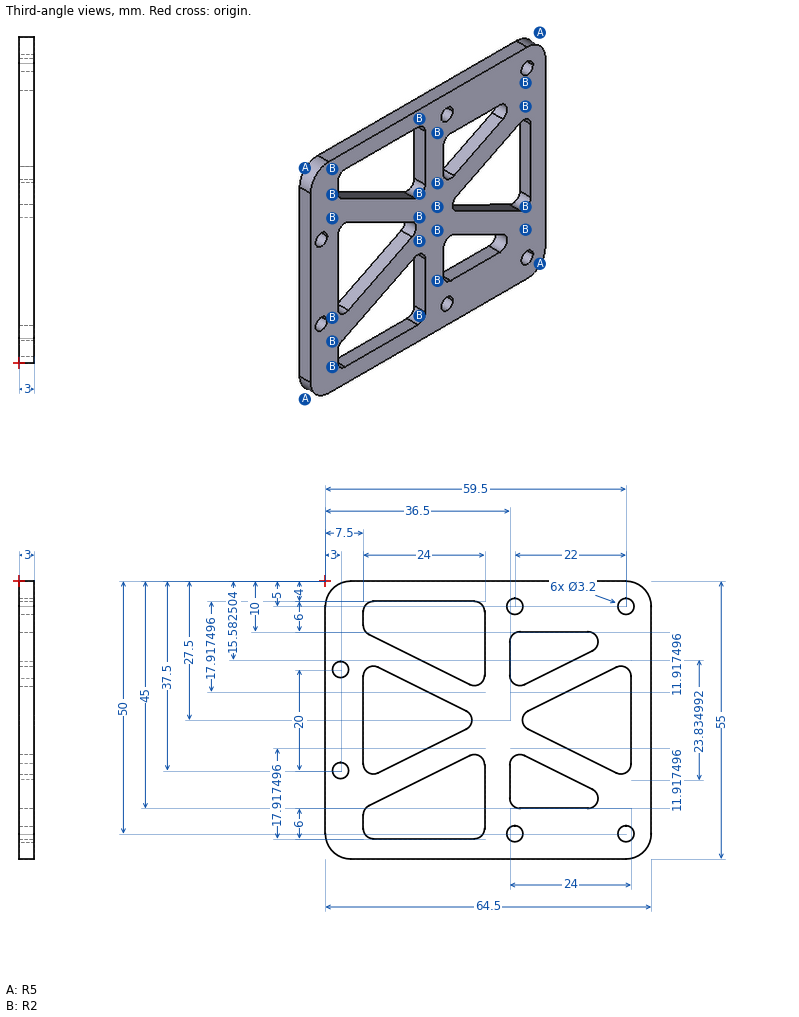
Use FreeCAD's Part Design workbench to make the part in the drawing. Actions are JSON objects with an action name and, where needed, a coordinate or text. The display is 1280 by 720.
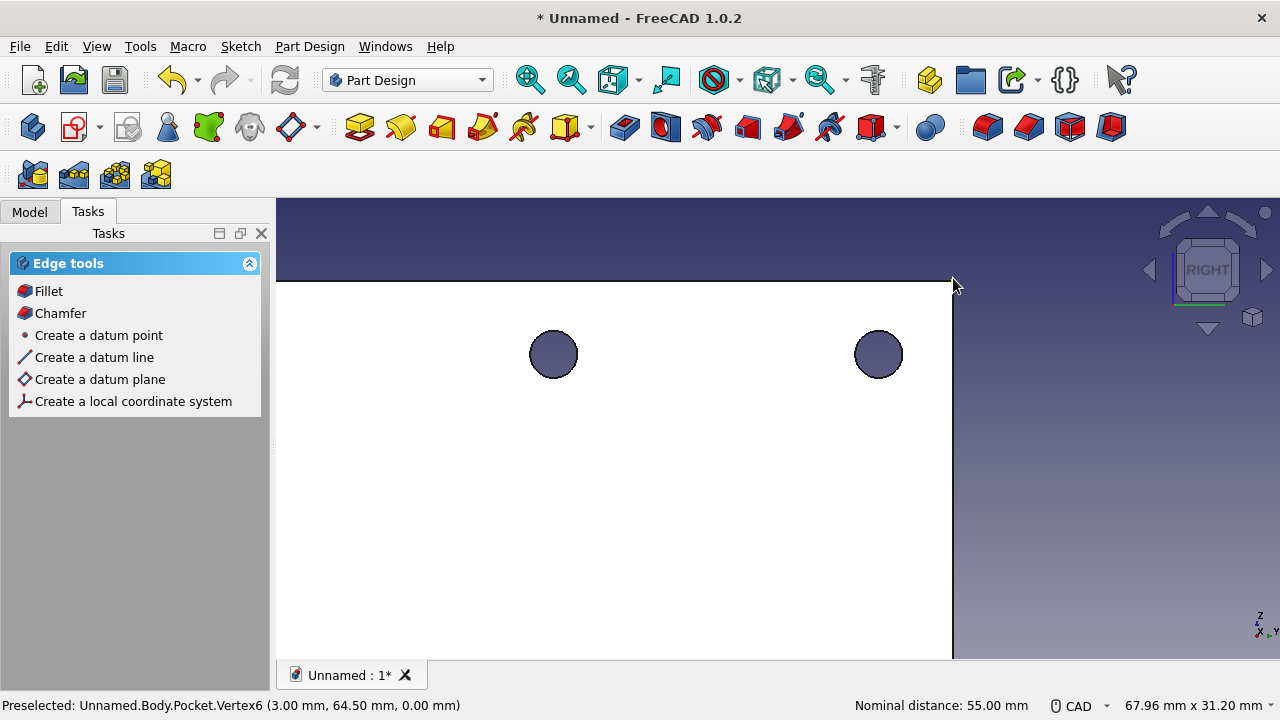
{"action": "left_click", "coordinate": [531, 80]}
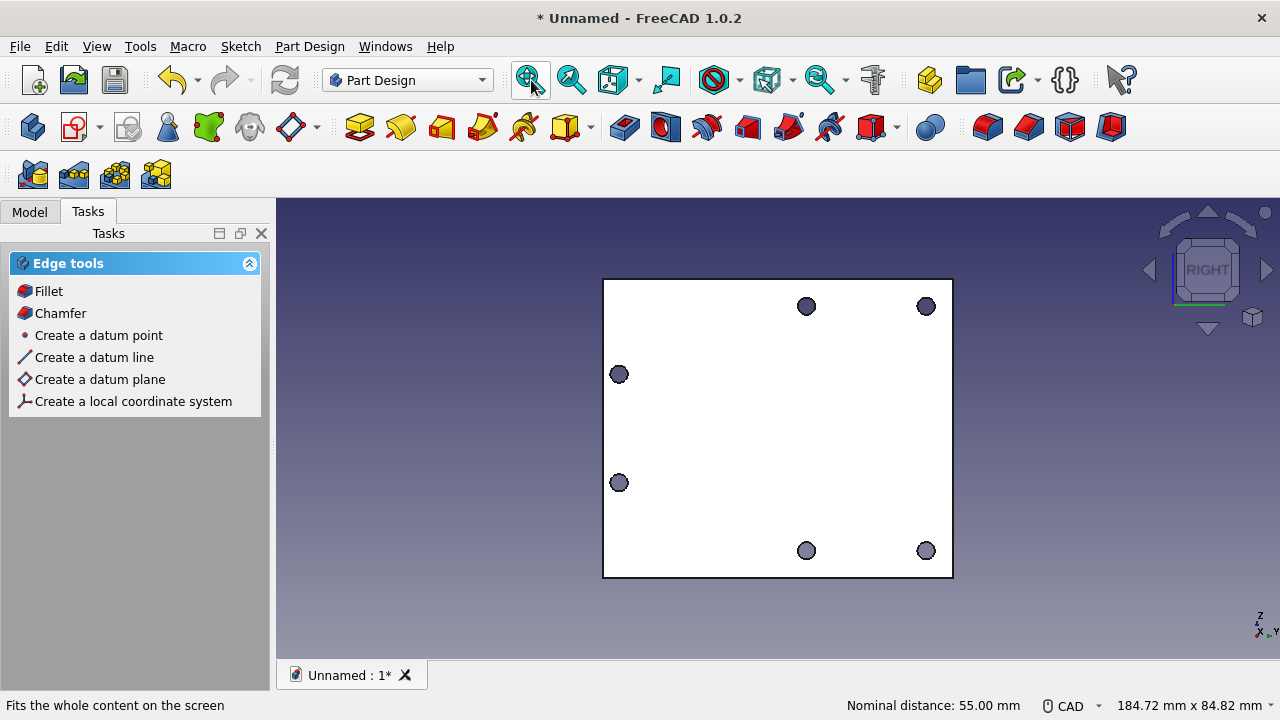
{"action": "key", "text": "5"}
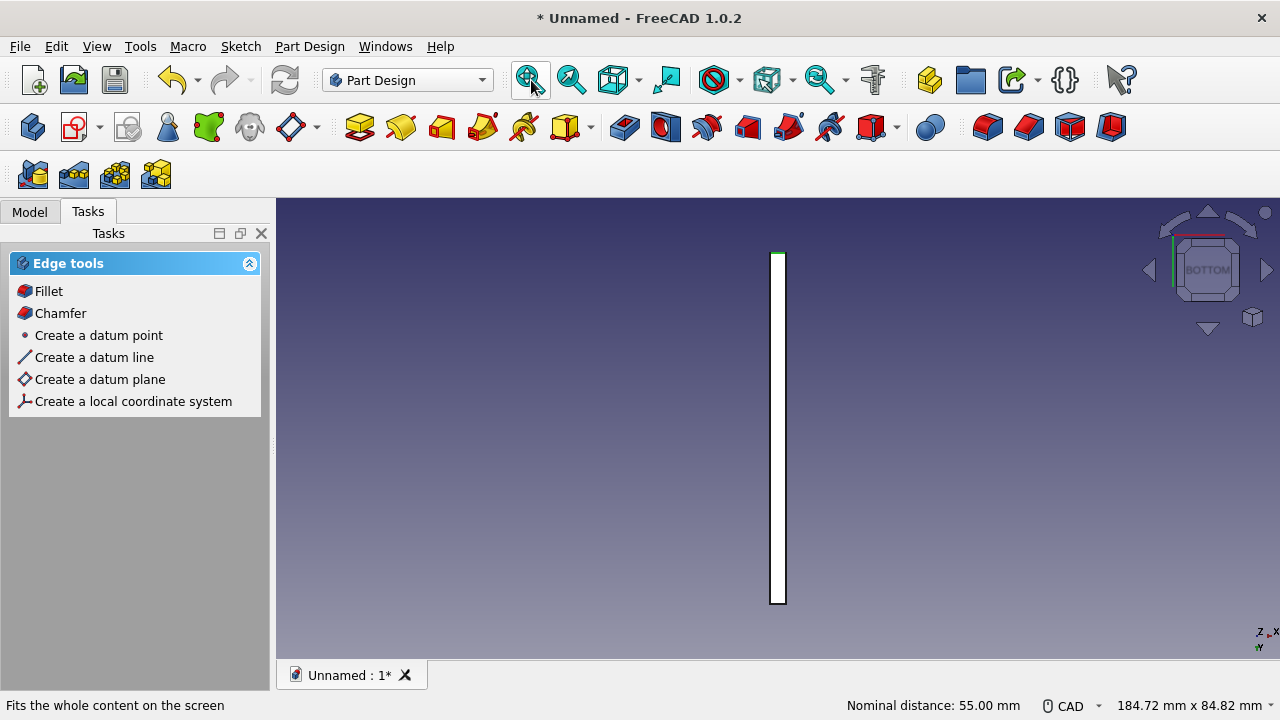
{"action": "left_click", "coordinate": [778, 603], "text": "ctrl"}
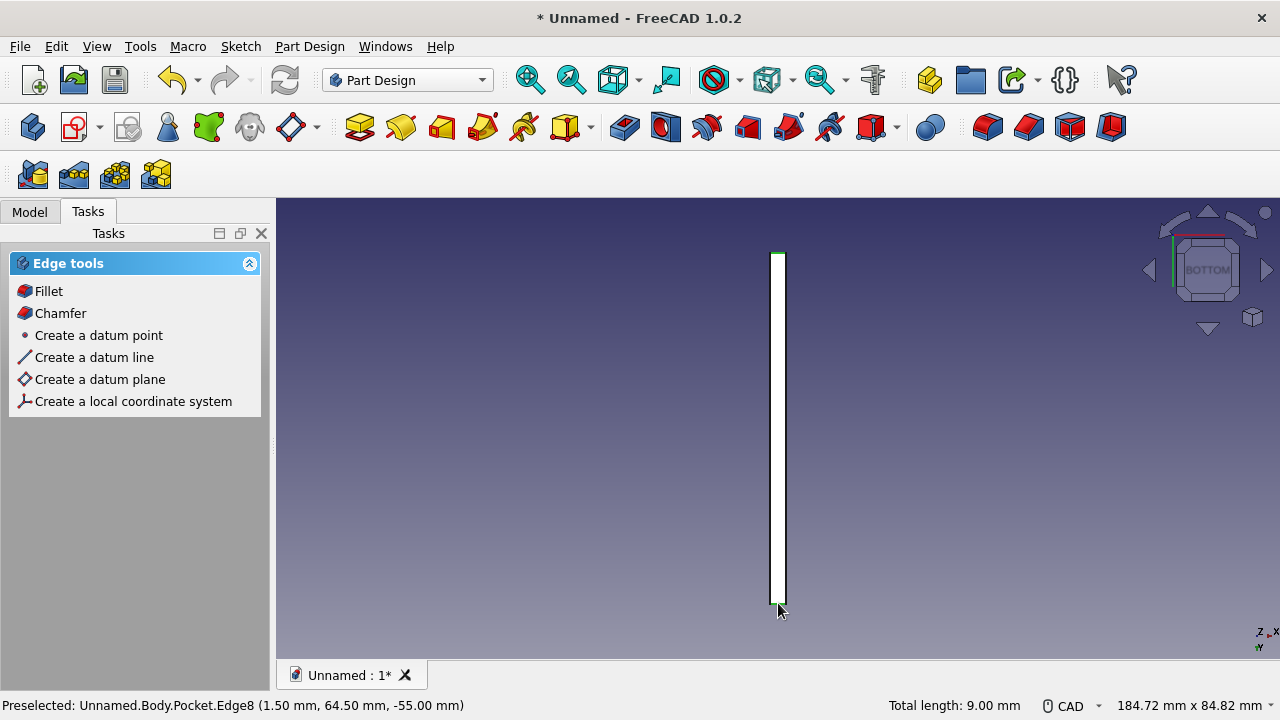
{"action": "scroll", "coordinate": [778, 603], "scroll_direction": "up", "scroll_amount": 5}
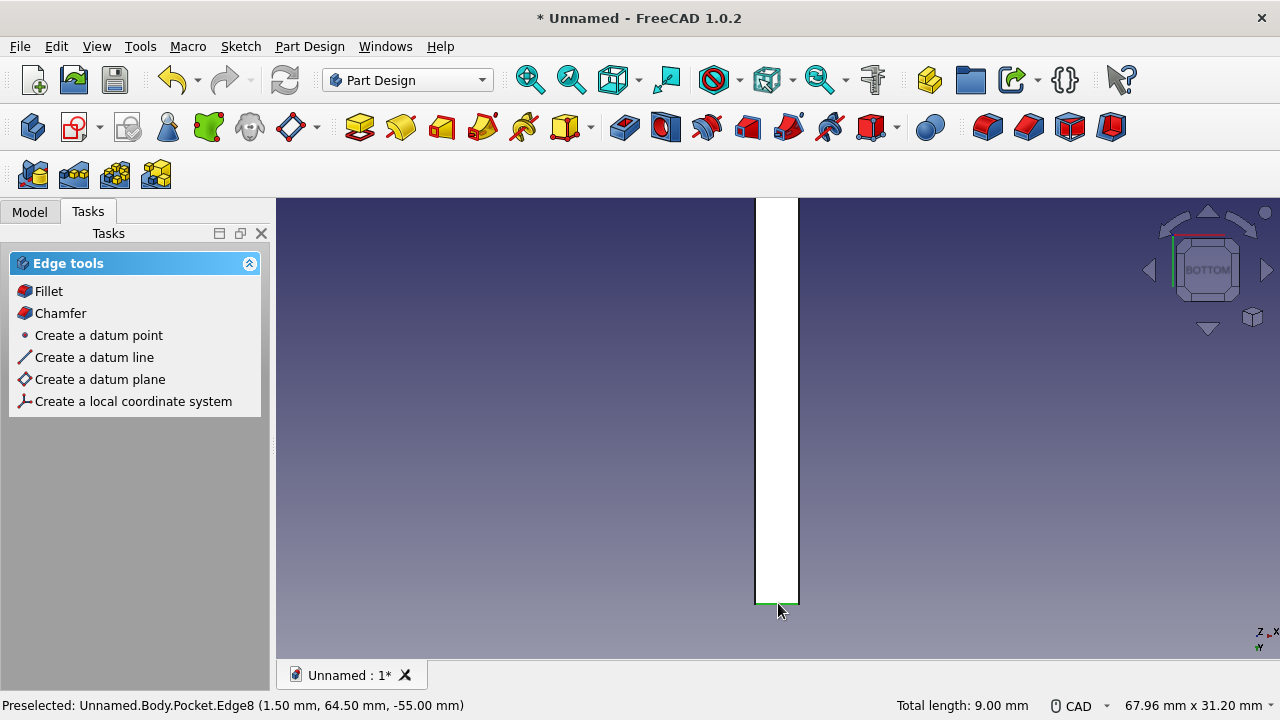
{"action": "left_click", "coordinate": [531, 80]}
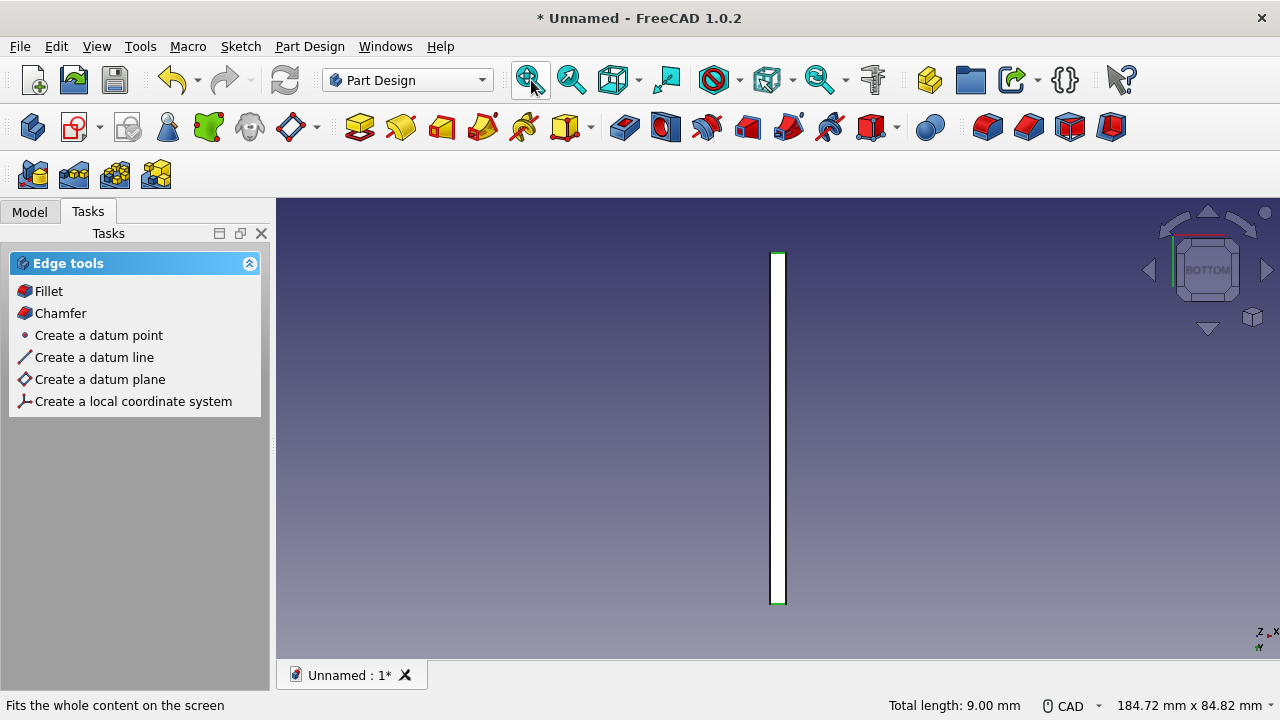
{"action": "key", "text": "4"}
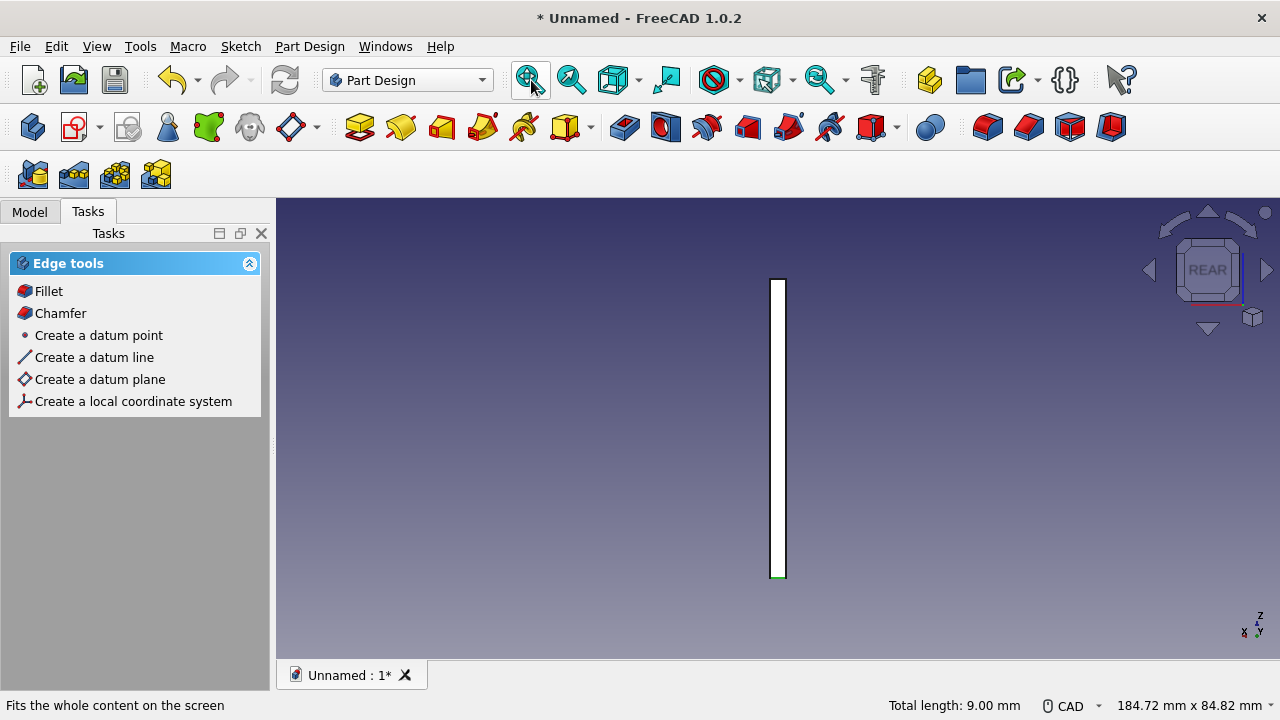
{"action": "left_click", "coordinate": [778, 278], "text": "ctrl"}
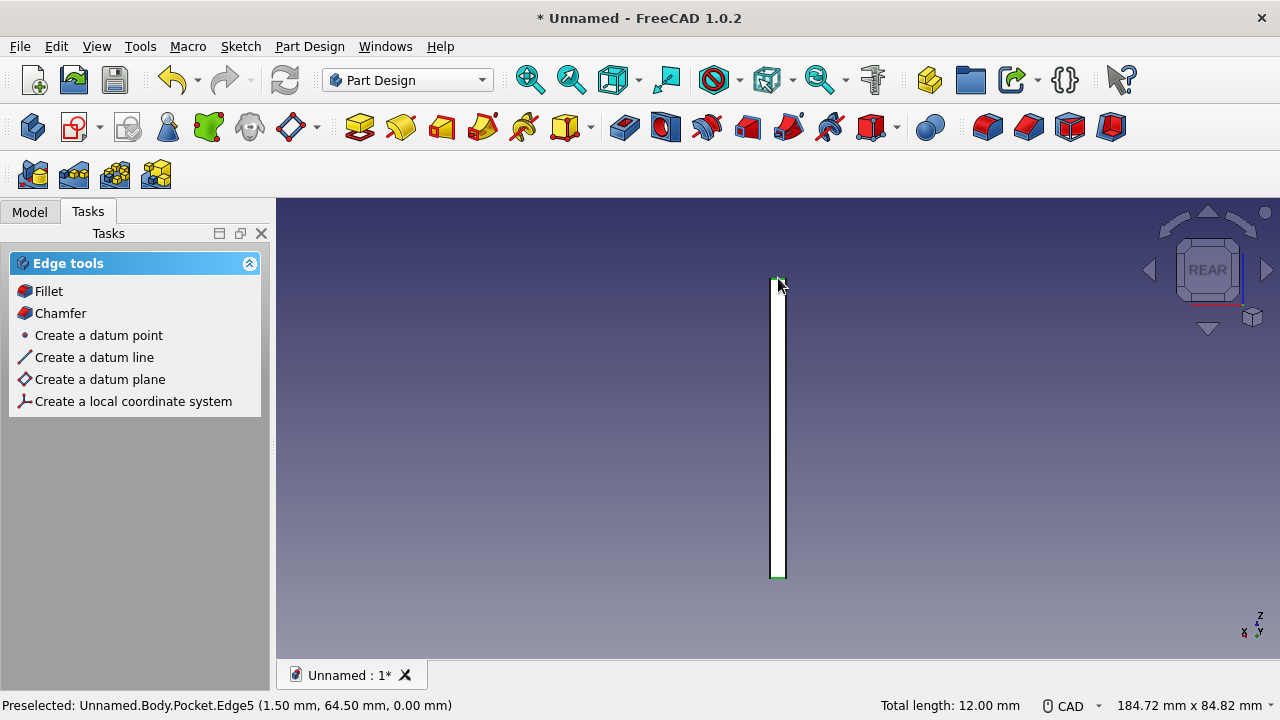
{"action": "left_click", "coordinate": [988, 128]}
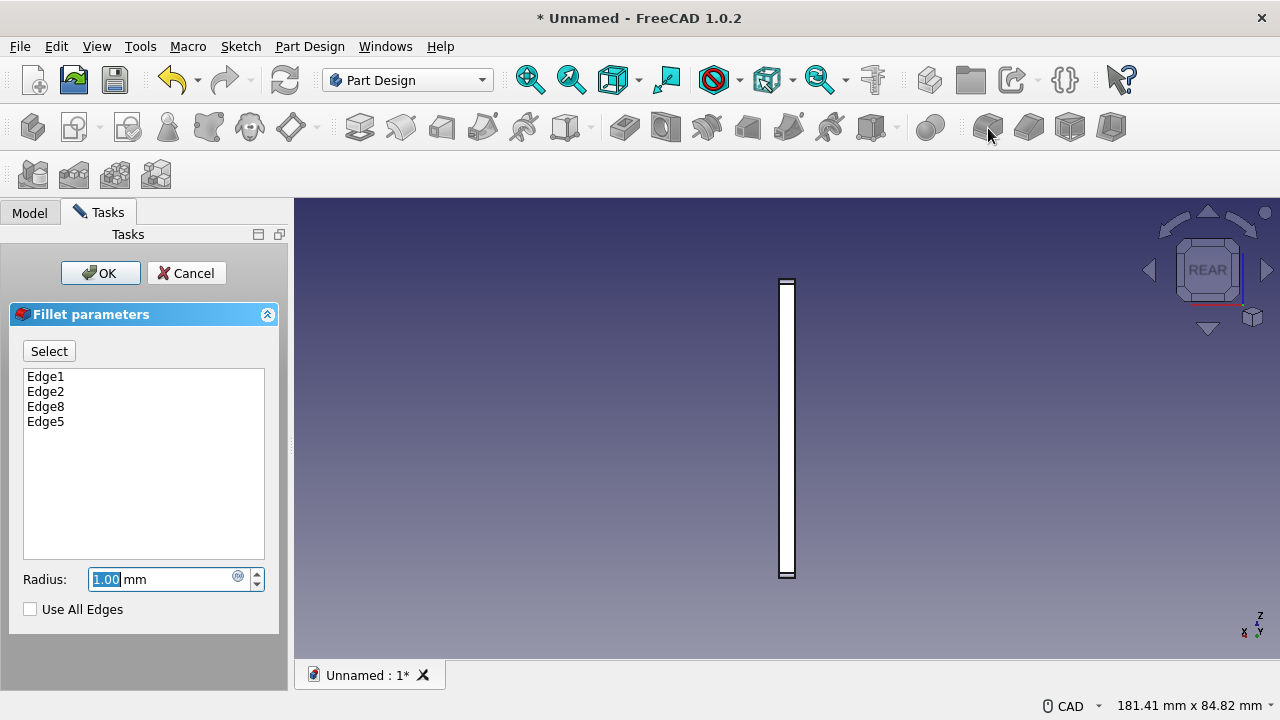
{"action": "type", "text": "5"}
{"action": "key", "text": "Tab"}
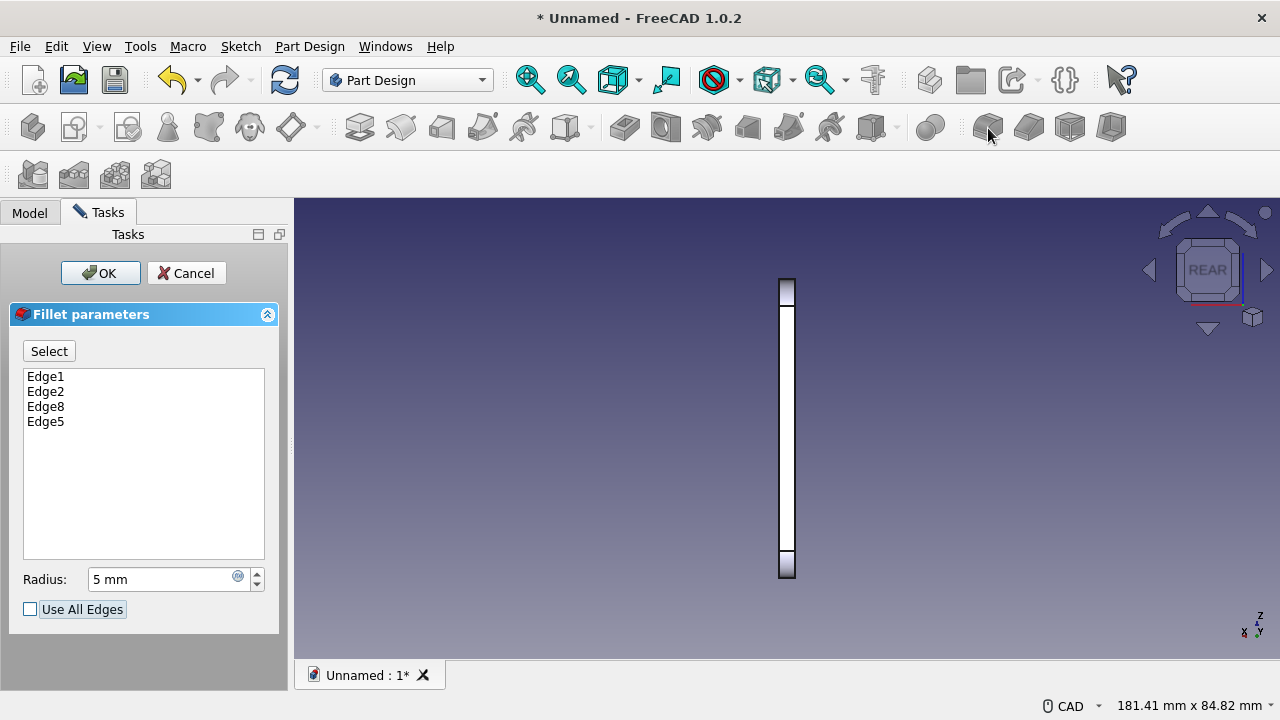
{"action": "left_click", "coordinate": [101, 273]}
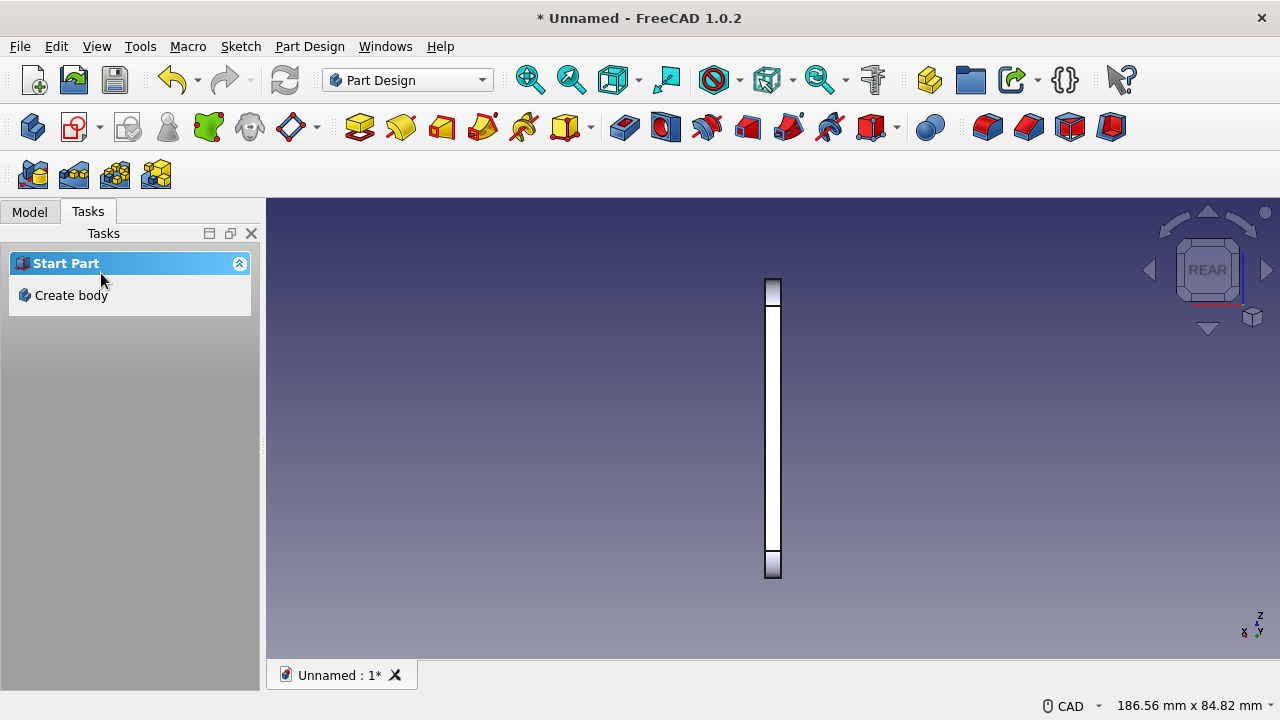
{"action": "left_click", "coordinate": [74, 128]}